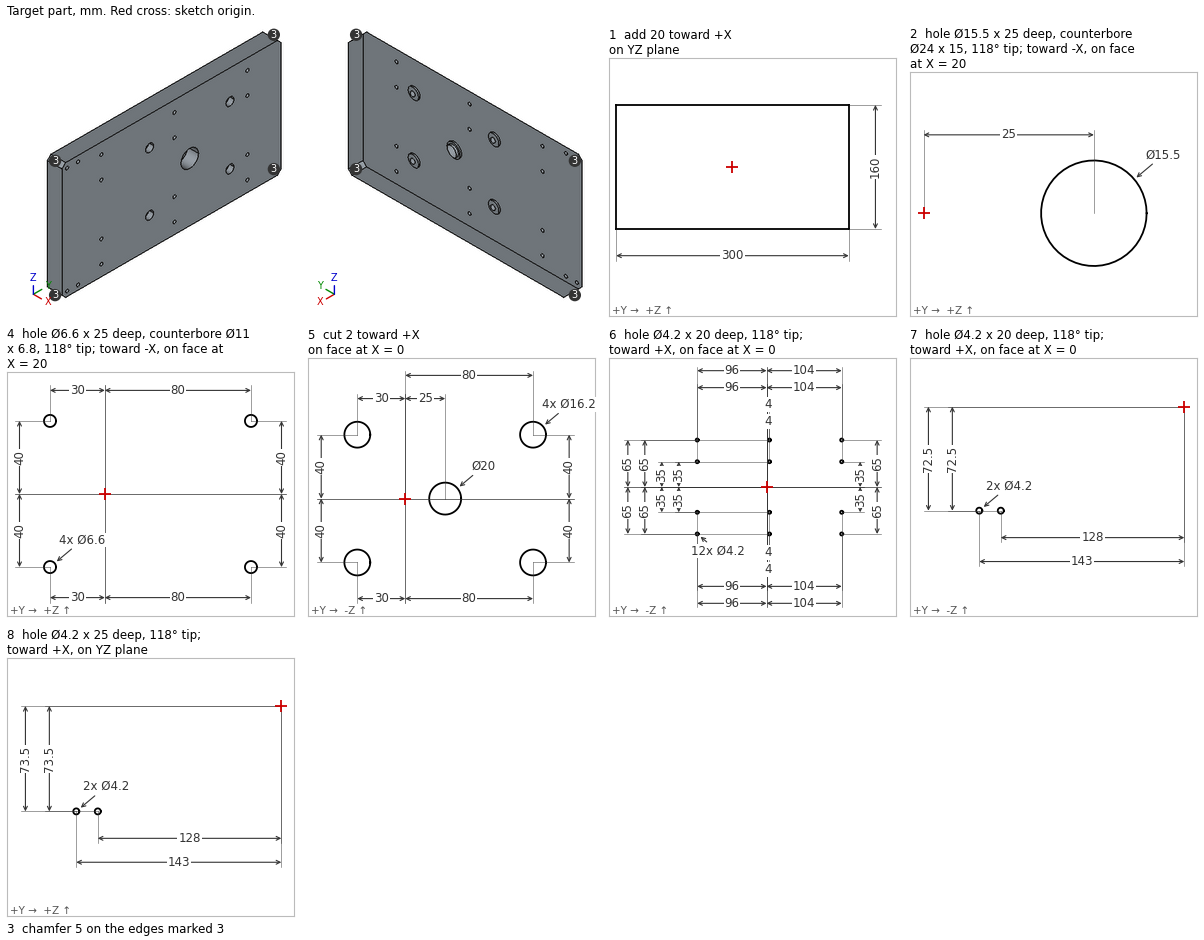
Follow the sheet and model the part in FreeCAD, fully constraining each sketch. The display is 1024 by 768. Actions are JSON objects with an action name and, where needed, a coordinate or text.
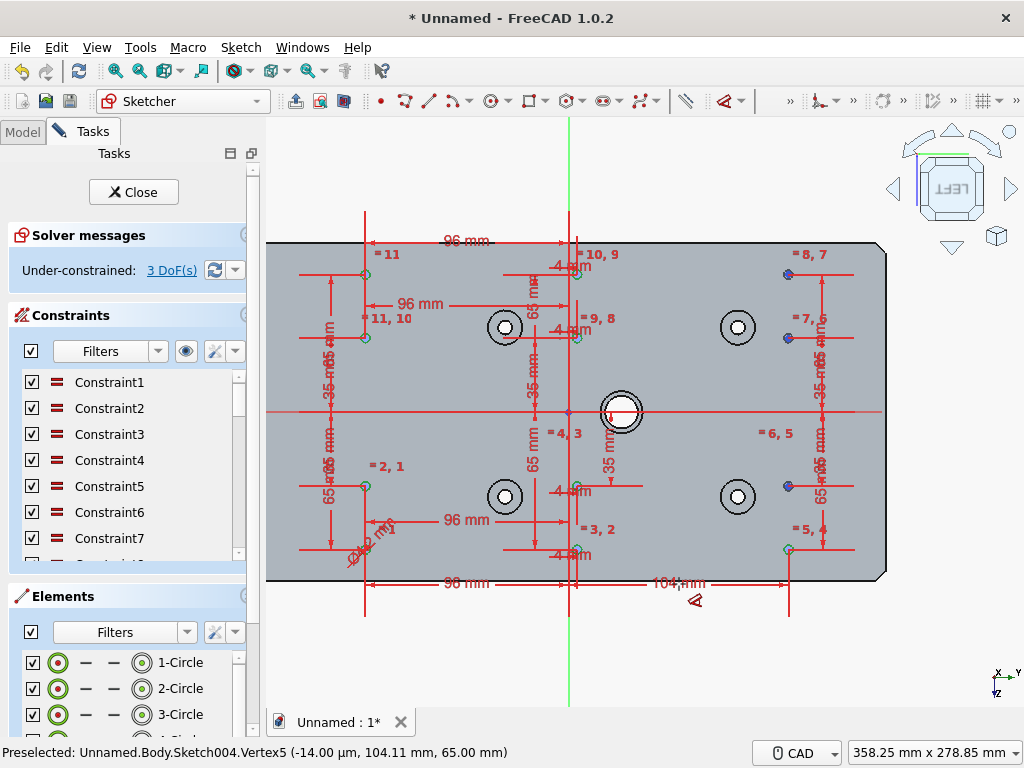
{"action": "left_click", "coordinate": [788, 486]}
{"action": "left_click", "coordinate": [678, 520]}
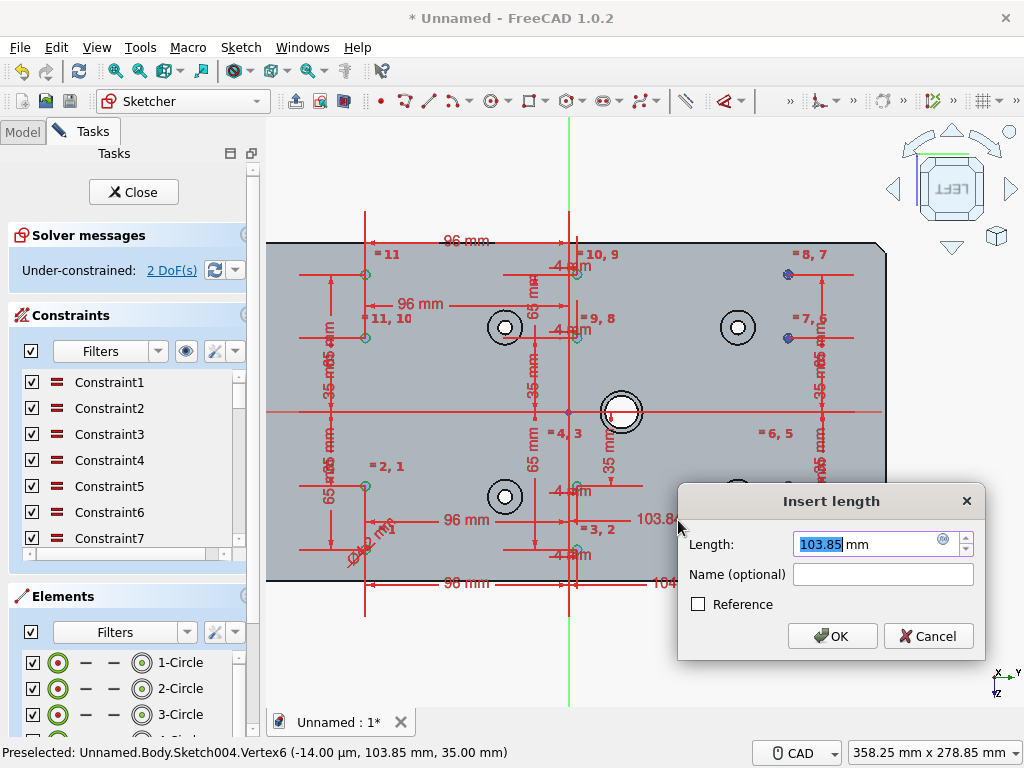
{"action": "type", "text": "104"}
{"action": "key", "text": "Return"}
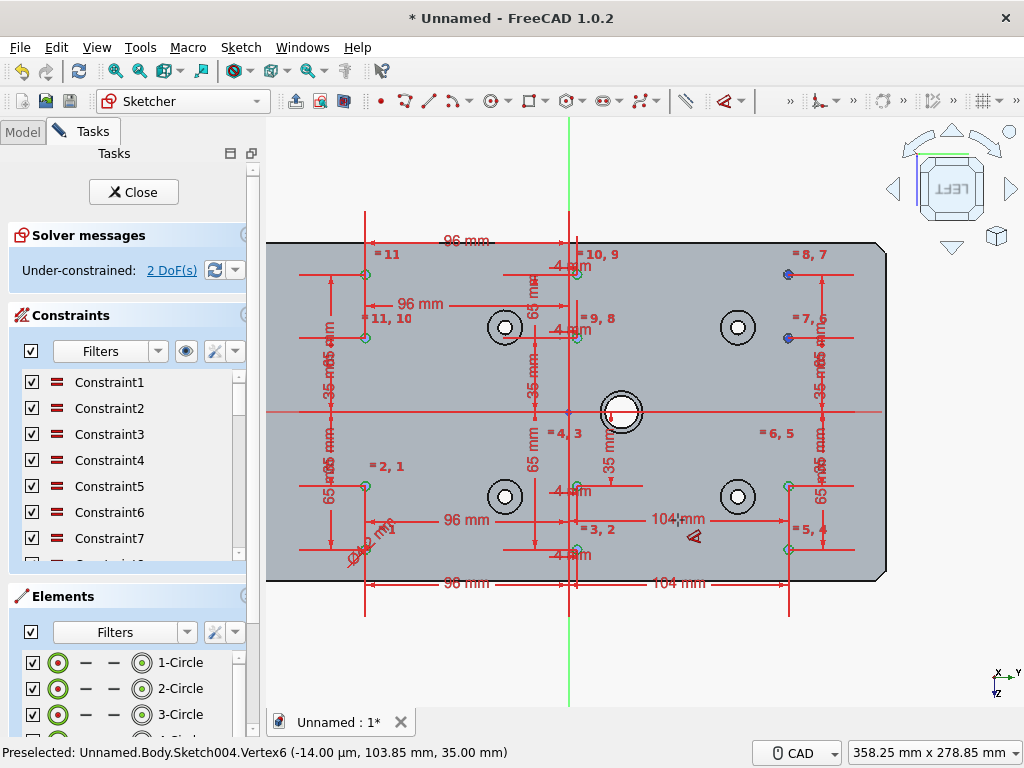
{"action": "left_click", "coordinate": [788, 338]}
{"action": "left_click", "coordinate": [678, 304]}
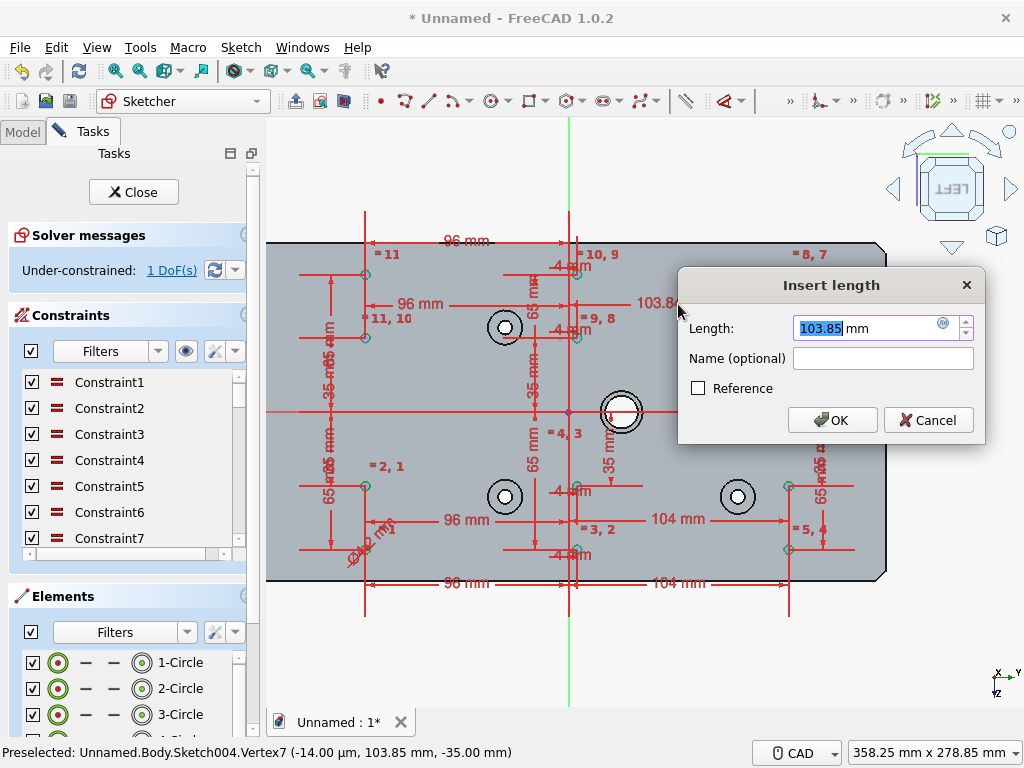
{"action": "type", "text": "104"}
{"action": "key", "text": "Return"}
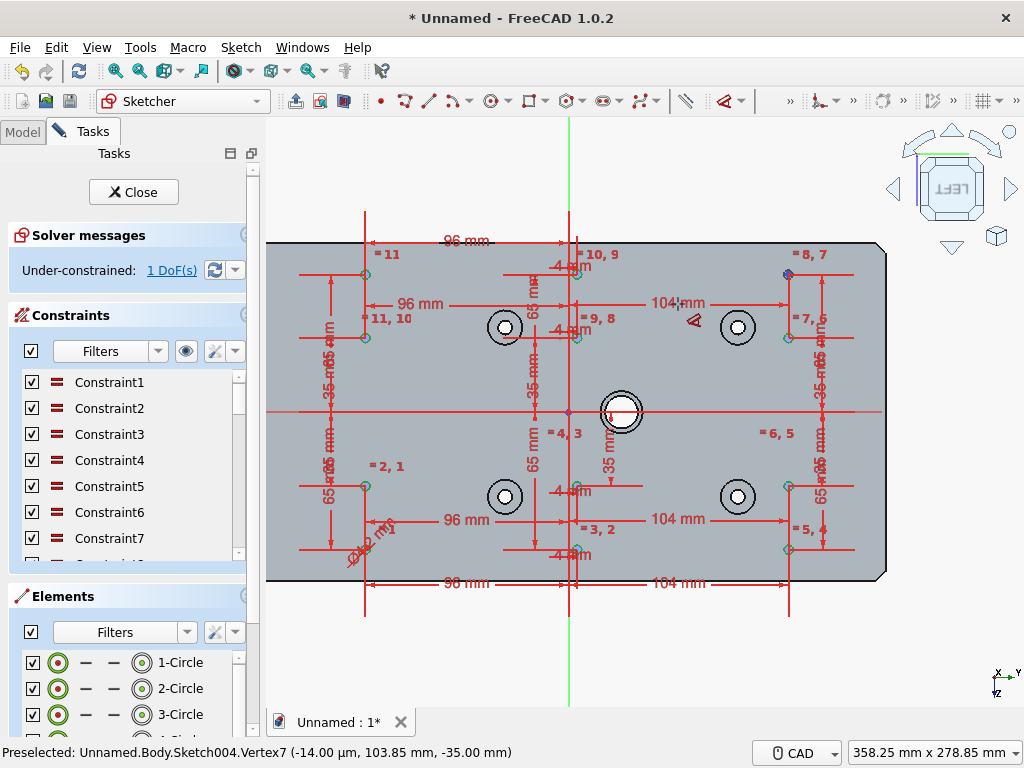
{"action": "left_click", "coordinate": [788, 275]}
{"action": "left_click", "coordinate": [678, 241]}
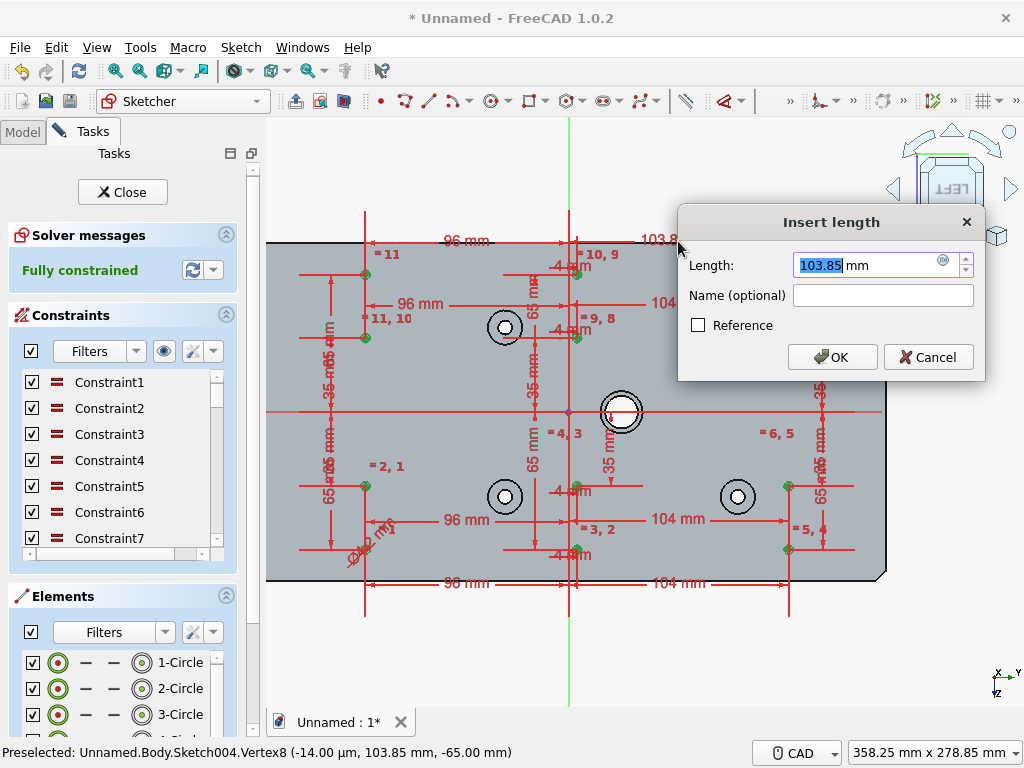
{"action": "type", "text": "104"}
{"action": "key", "text": "Return"}
{"action": "key", "text": "Escape"}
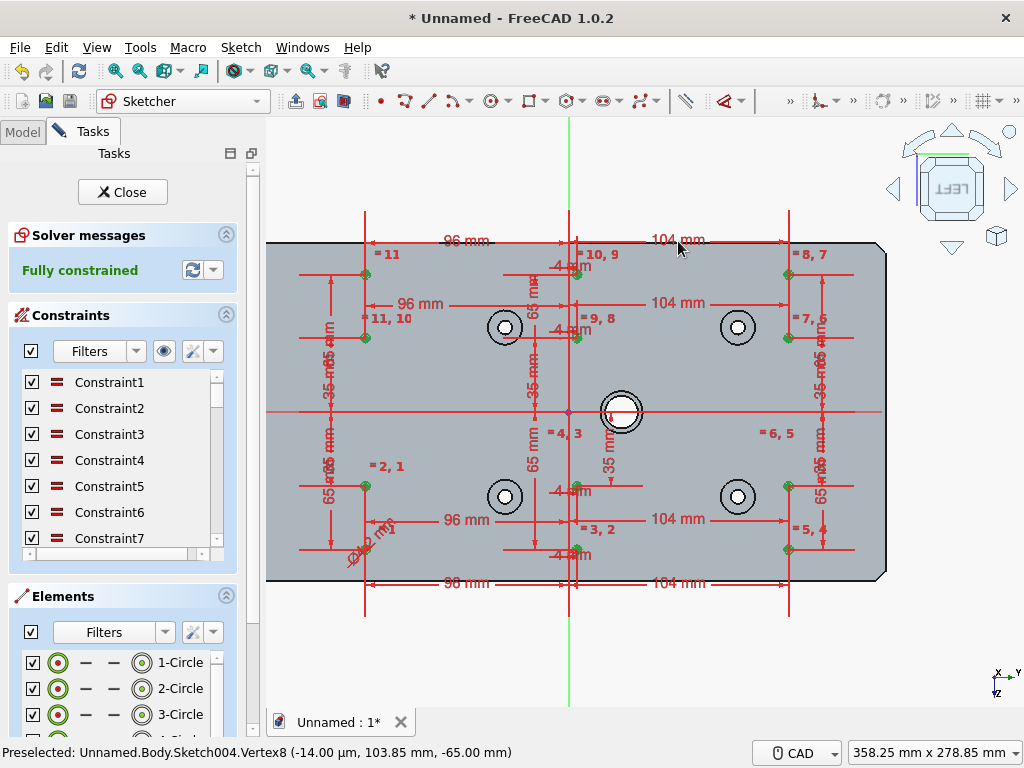
{"action": "left_click", "coordinate": [123, 192]}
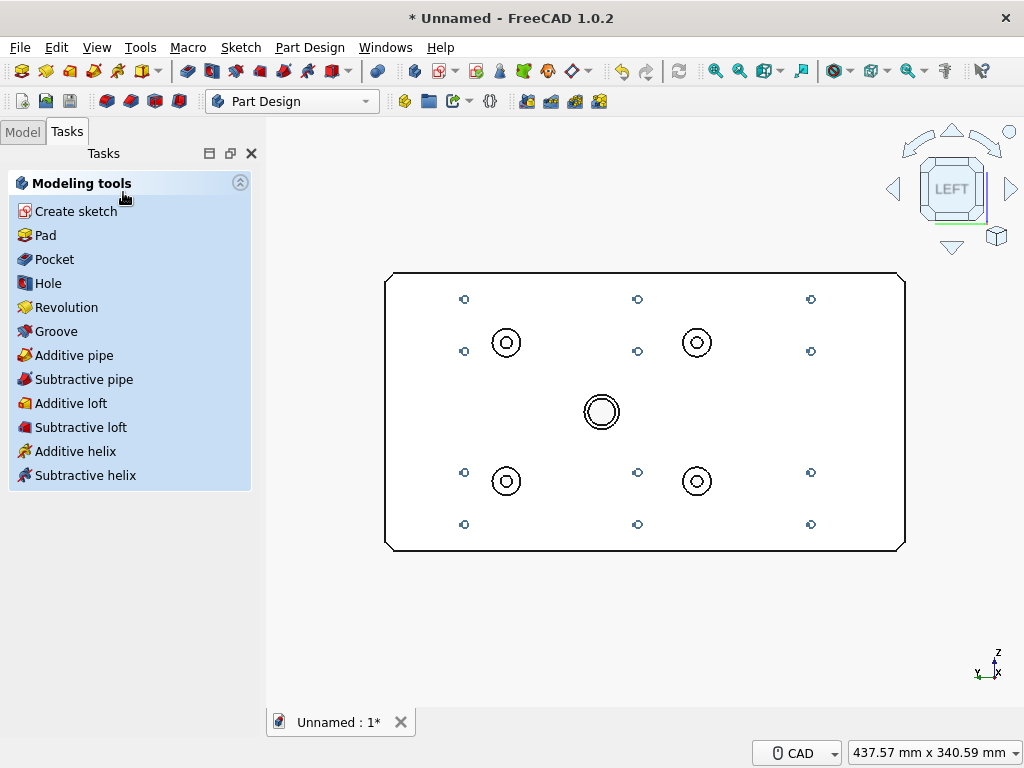
{"action": "left_click", "coordinate": [212, 72]}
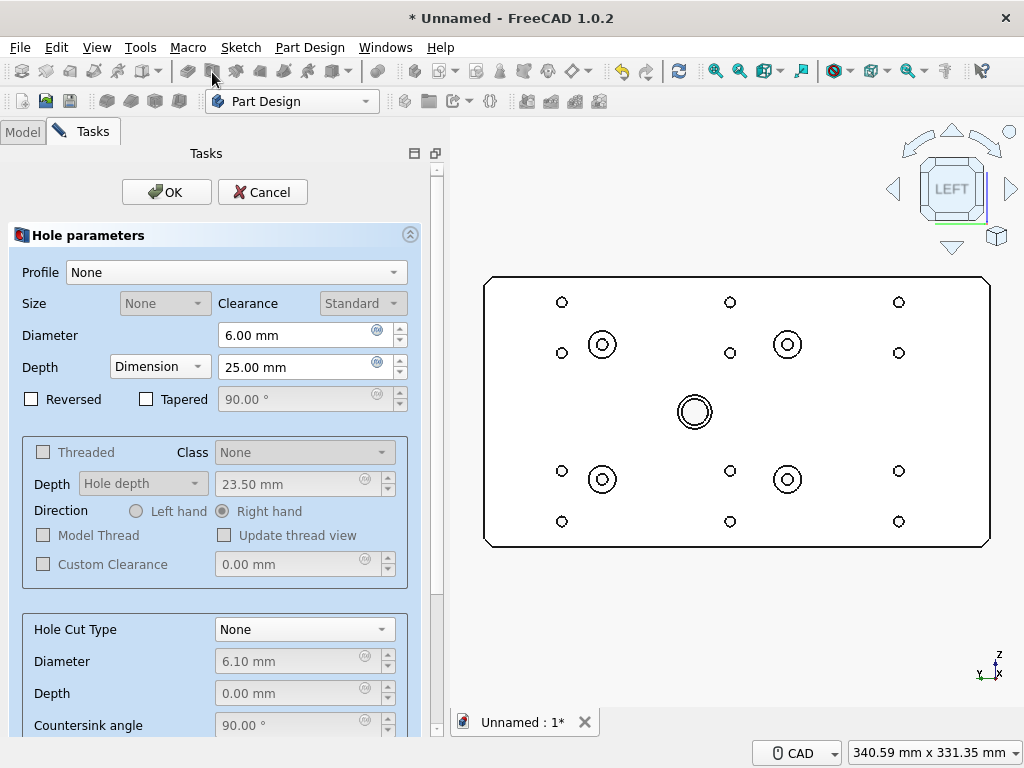
{"action": "triple_click", "coordinate": [305, 335]}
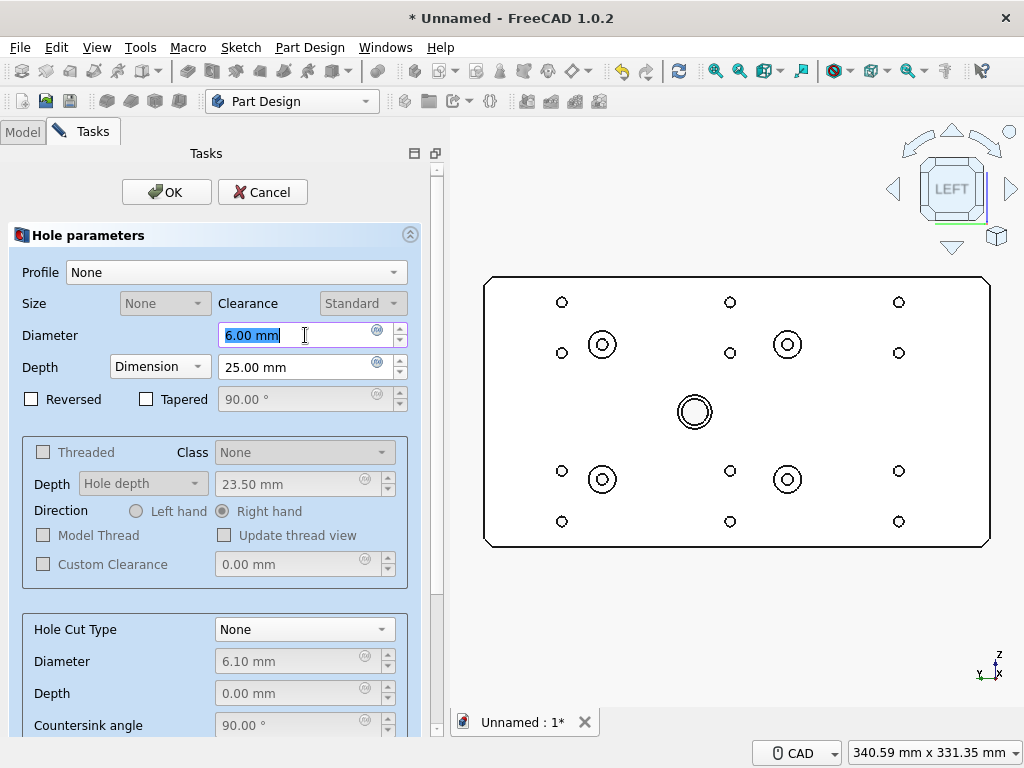
{"action": "type", "text": "4.2"}
{"action": "key", "text": "Tab"}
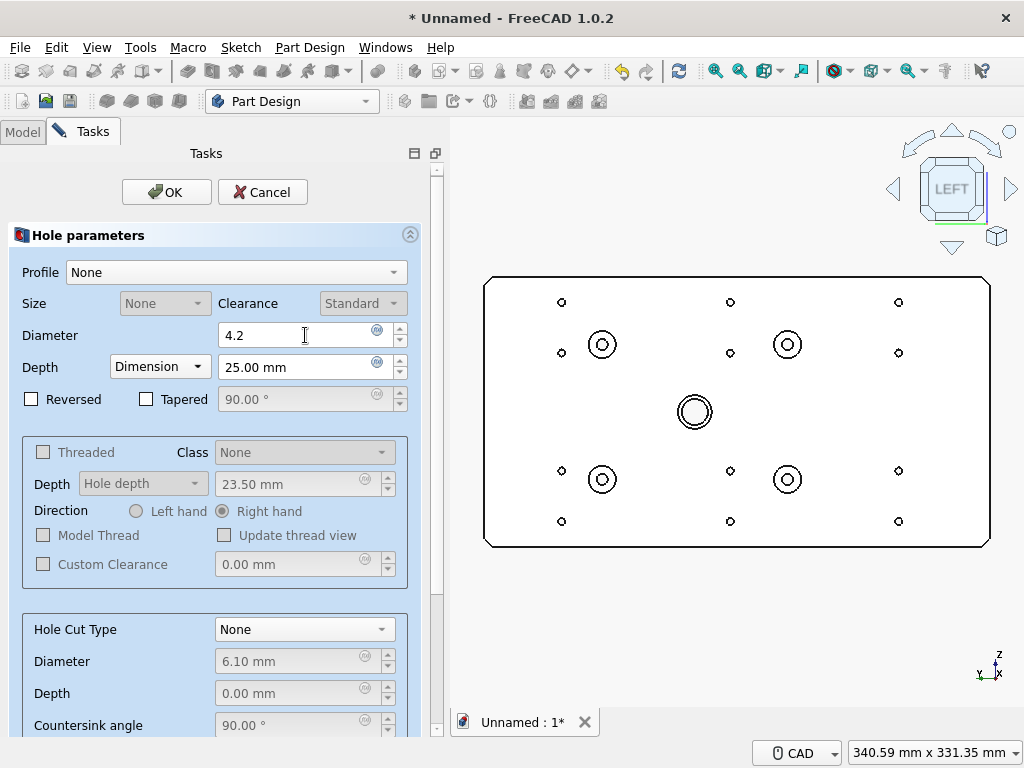
{"action": "triple_click", "coordinate": [305, 367]}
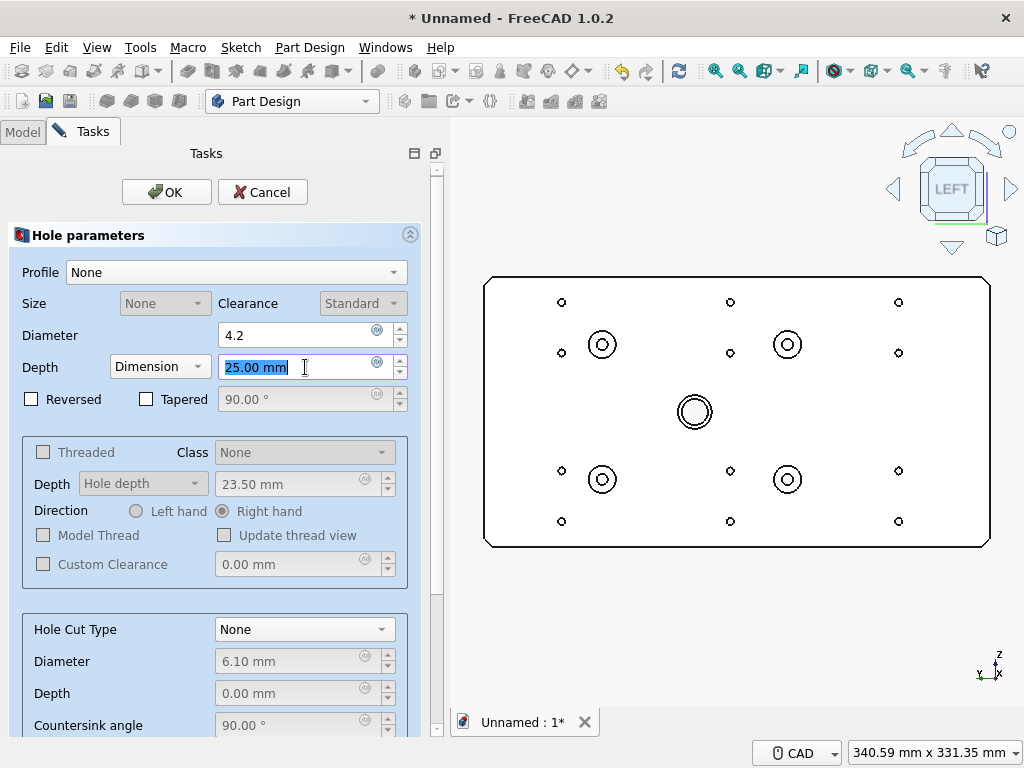
{"action": "type", "text": "20"}
{"action": "key", "text": "Tab"}